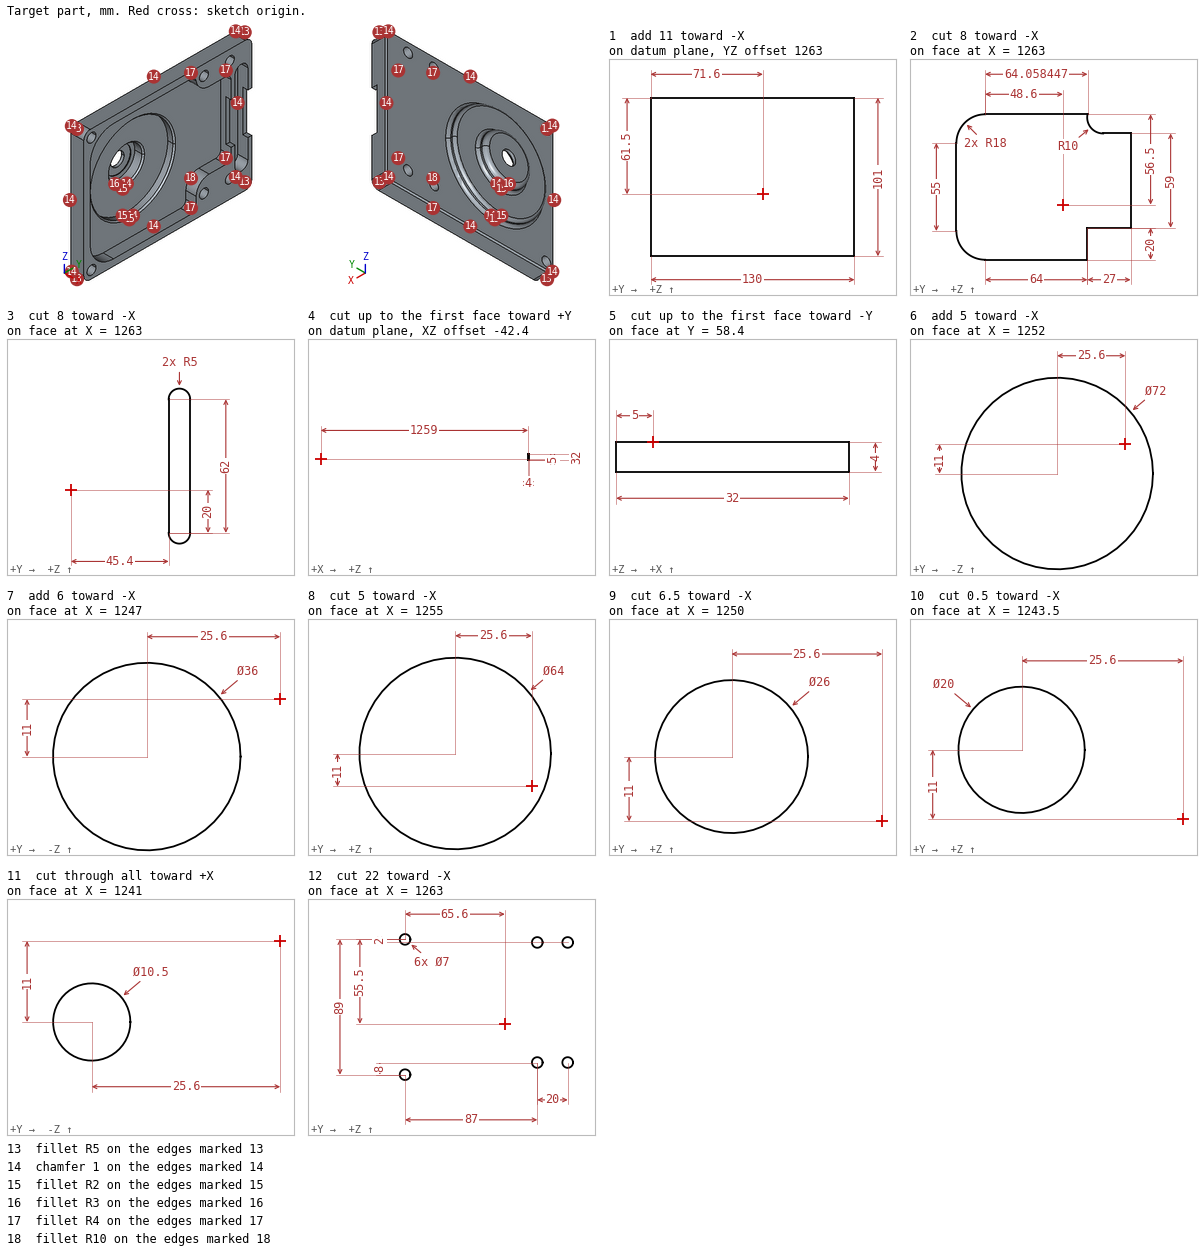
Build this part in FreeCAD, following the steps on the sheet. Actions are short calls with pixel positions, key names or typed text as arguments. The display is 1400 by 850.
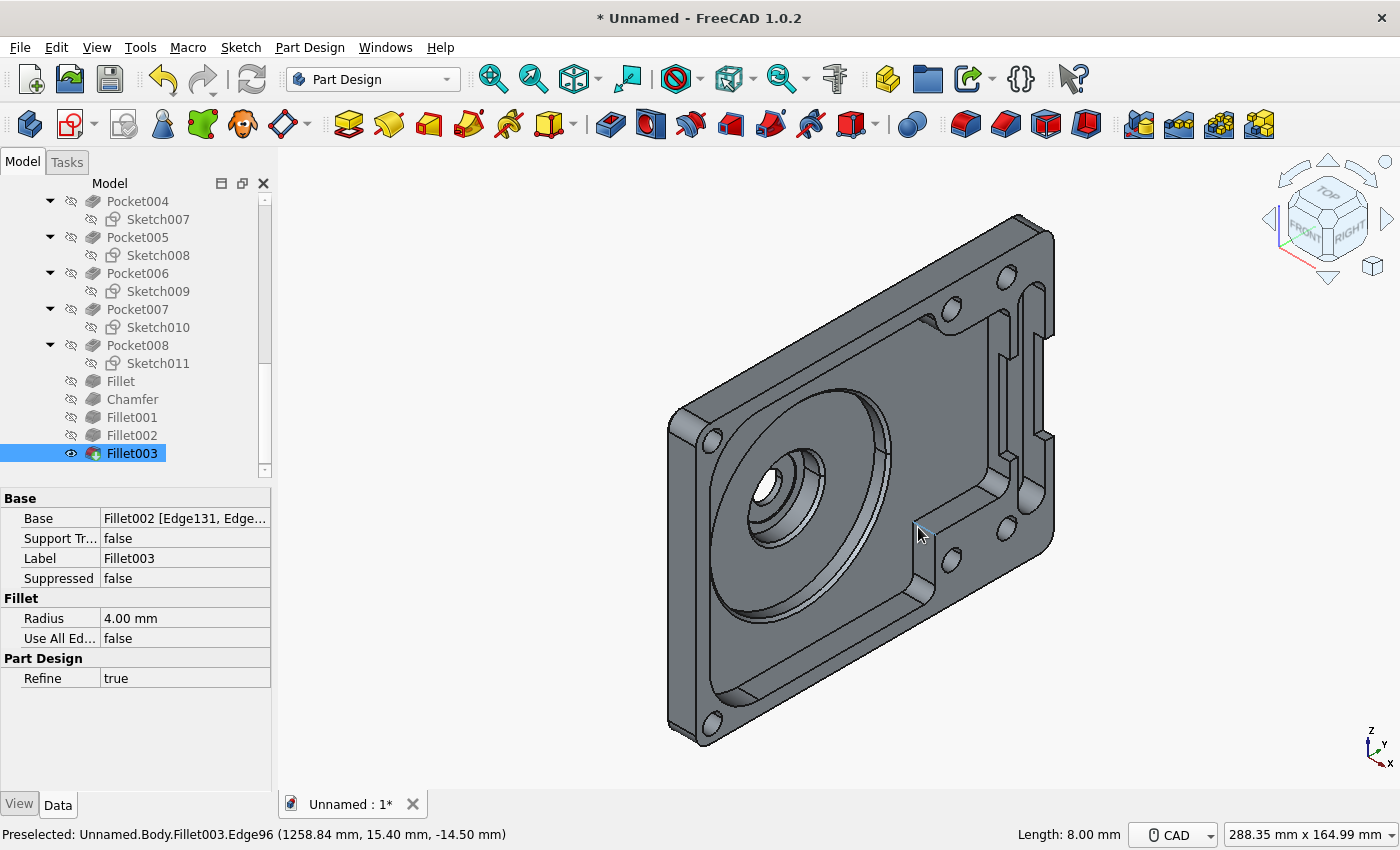
click(966, 124)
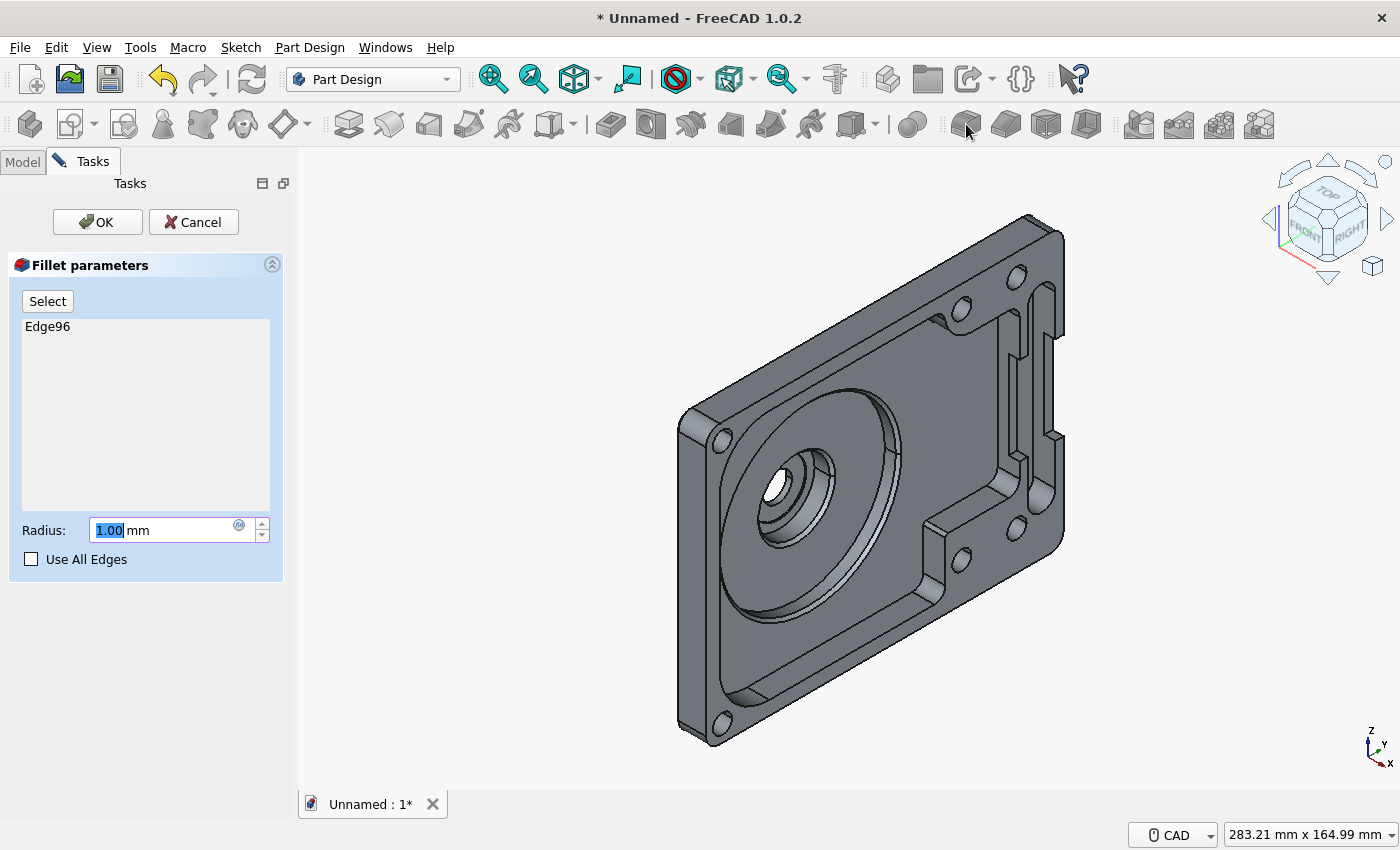
text(10)
key(Tab)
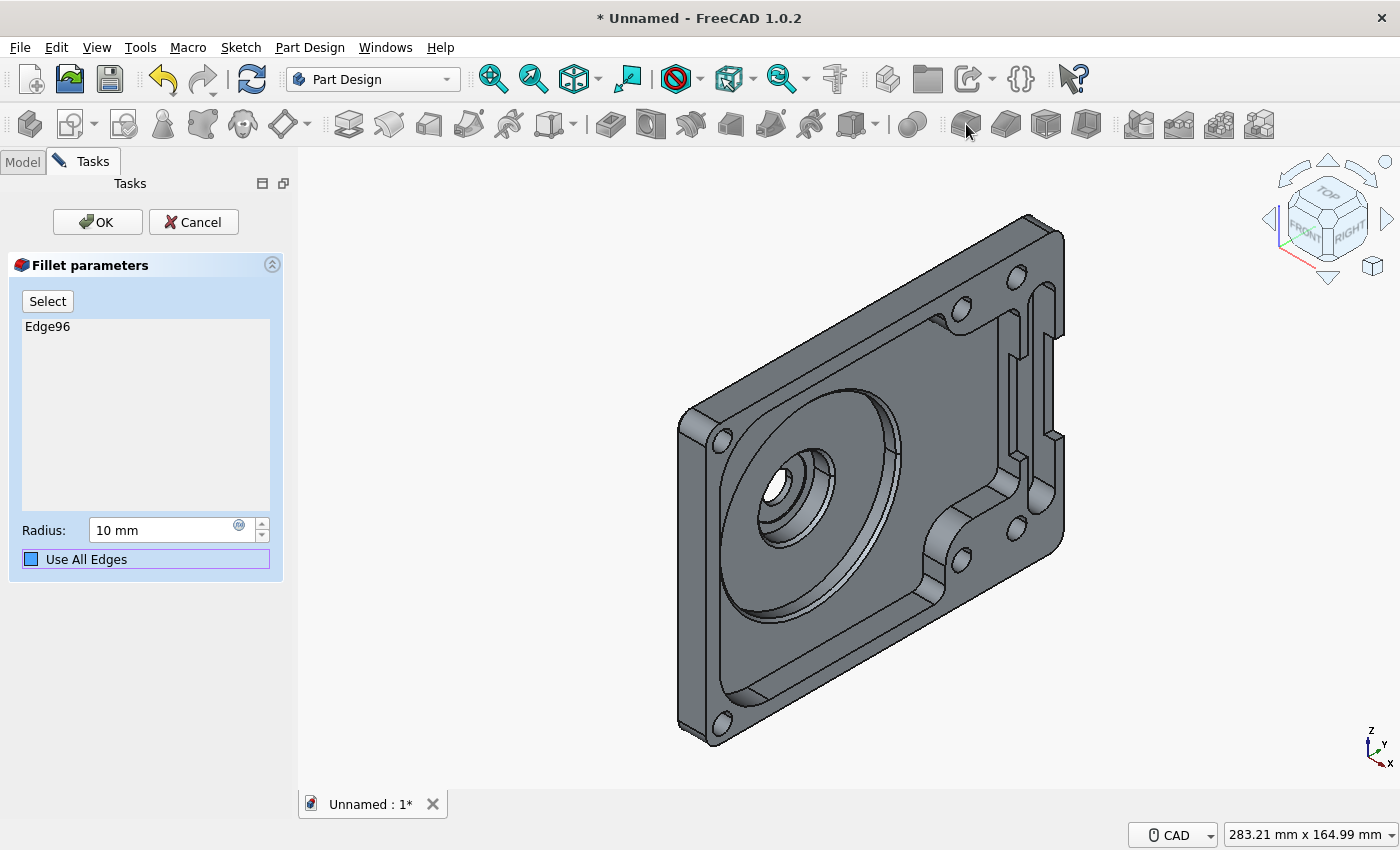
click(98, 222)